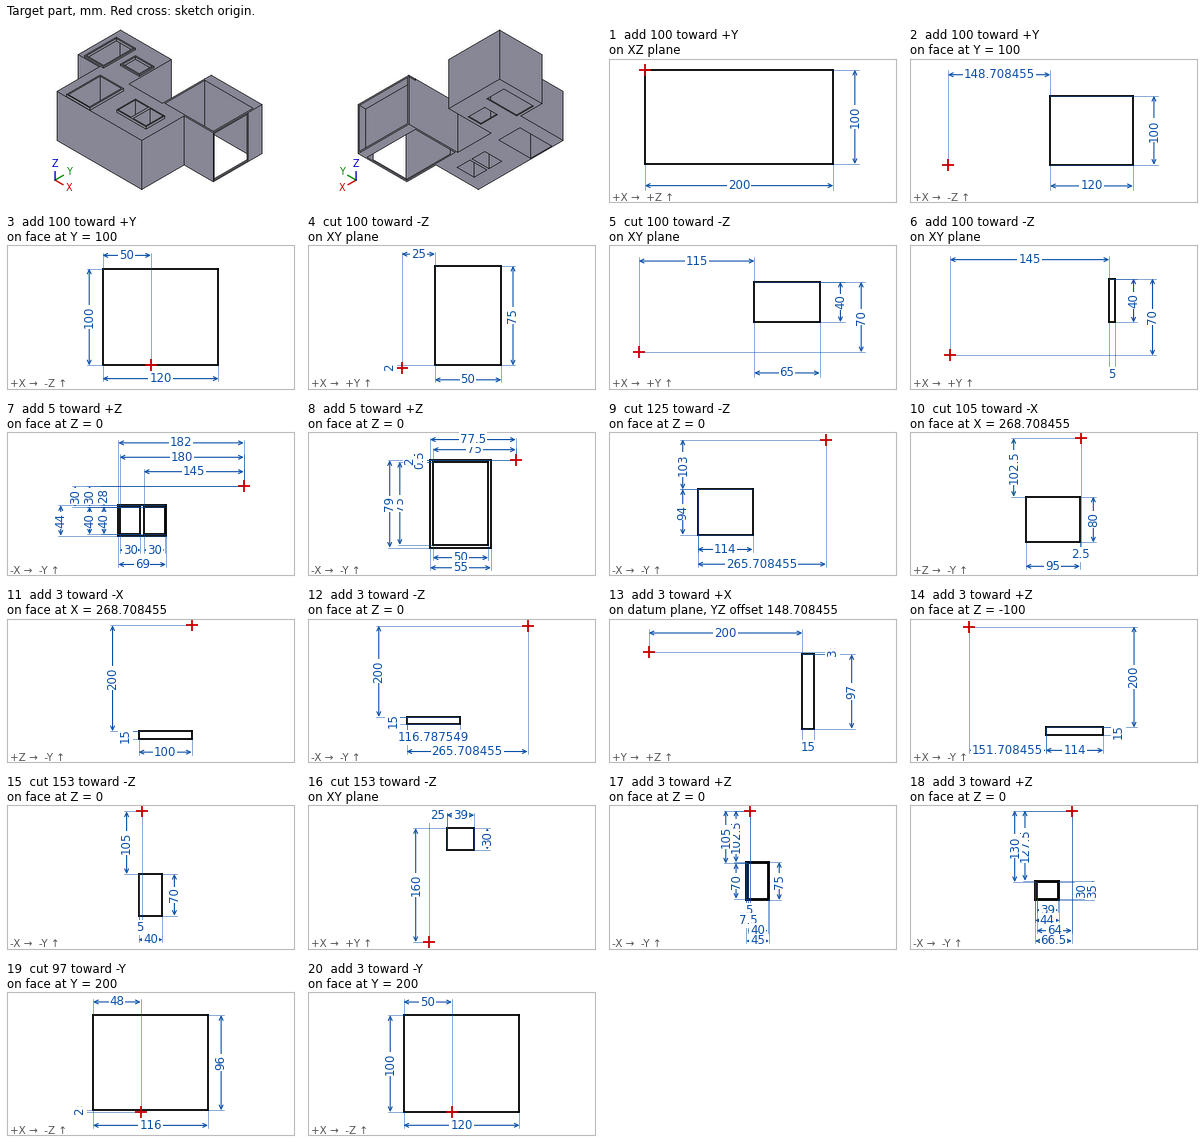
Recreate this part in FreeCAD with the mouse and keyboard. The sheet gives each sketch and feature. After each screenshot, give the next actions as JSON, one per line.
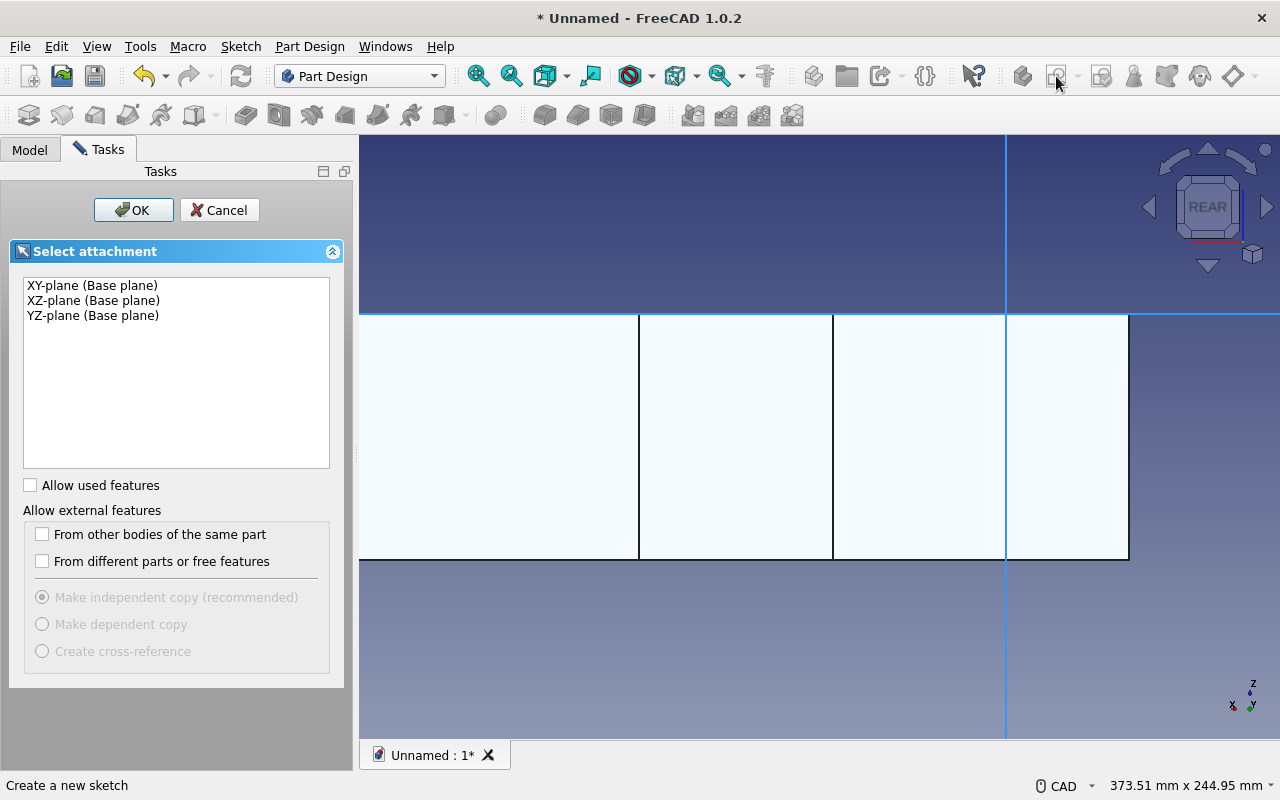
{"action": "left_click", "coordinate": [84, 286]}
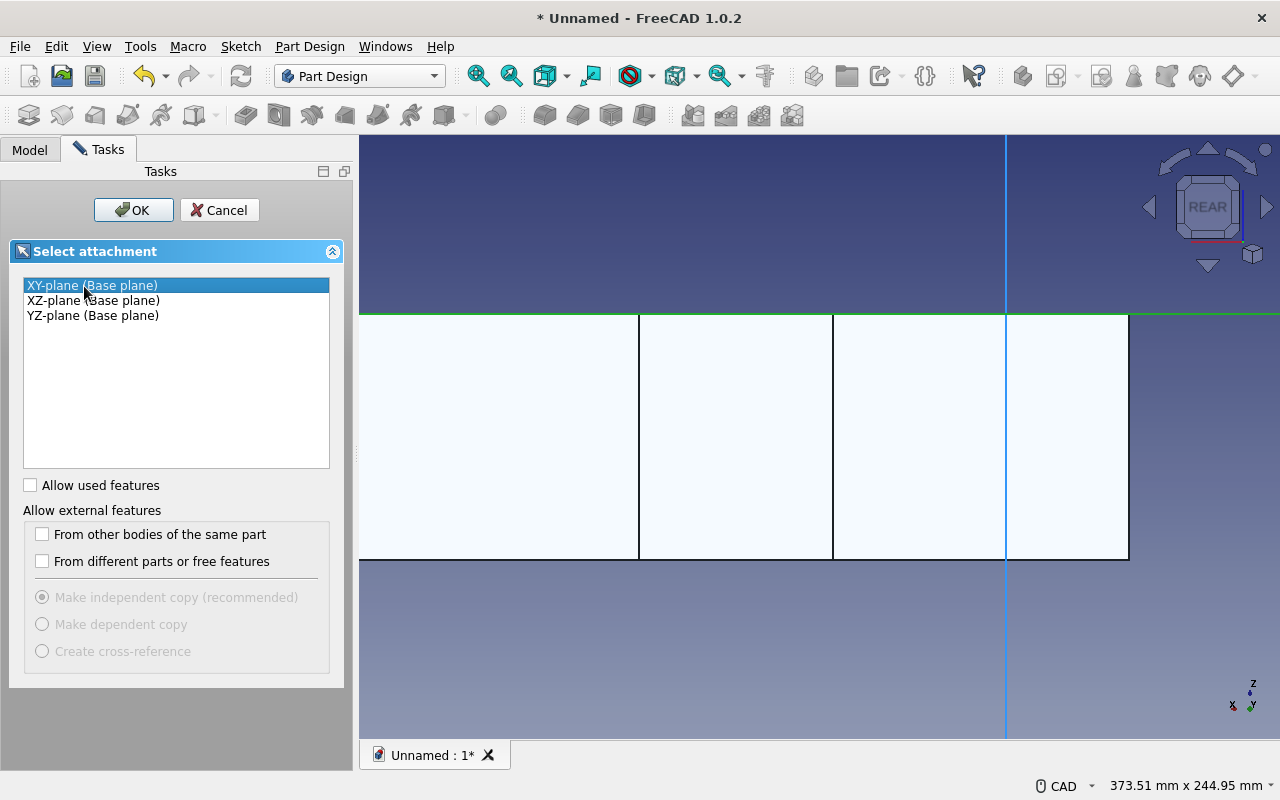
{"action": "left_click", "coordinate": [134, 210]}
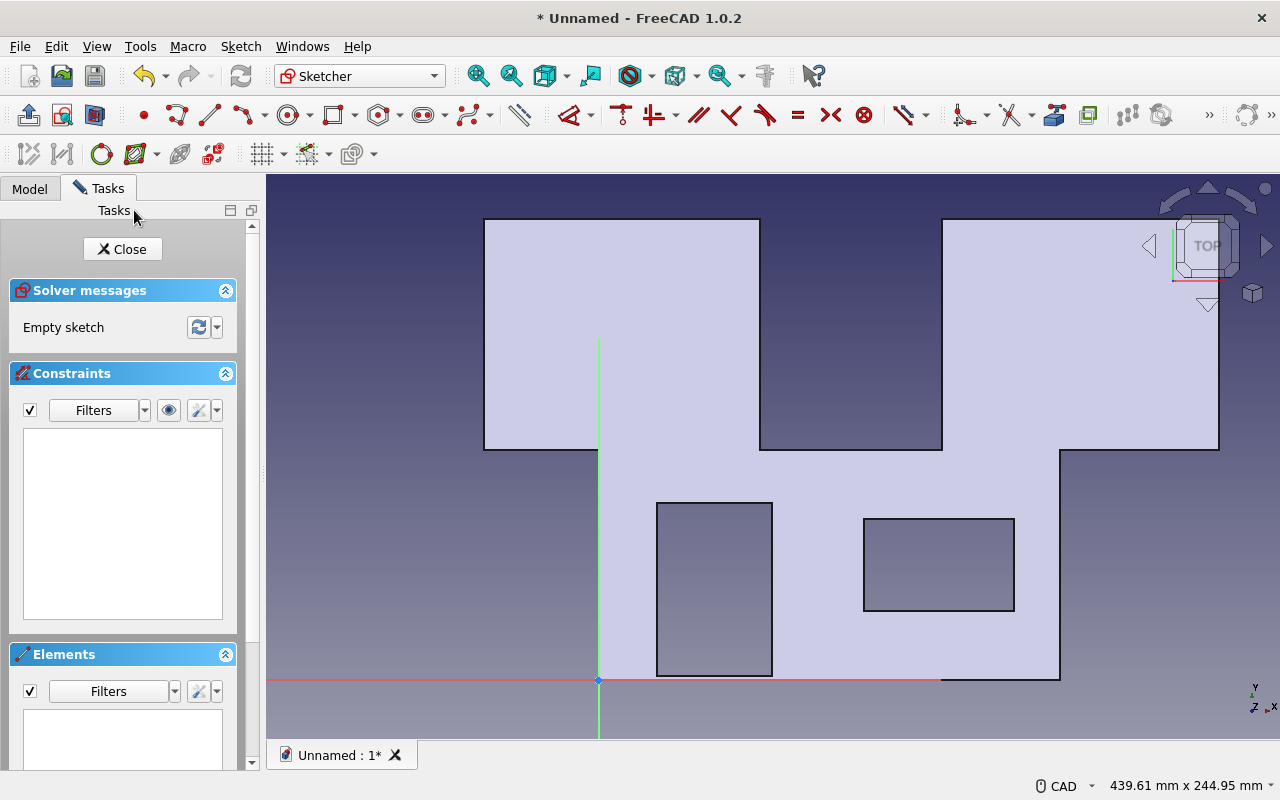
{"action": "scroll", "coordinate": [1016, 600], "scroll_direction": "up", "scroll_amount": 7}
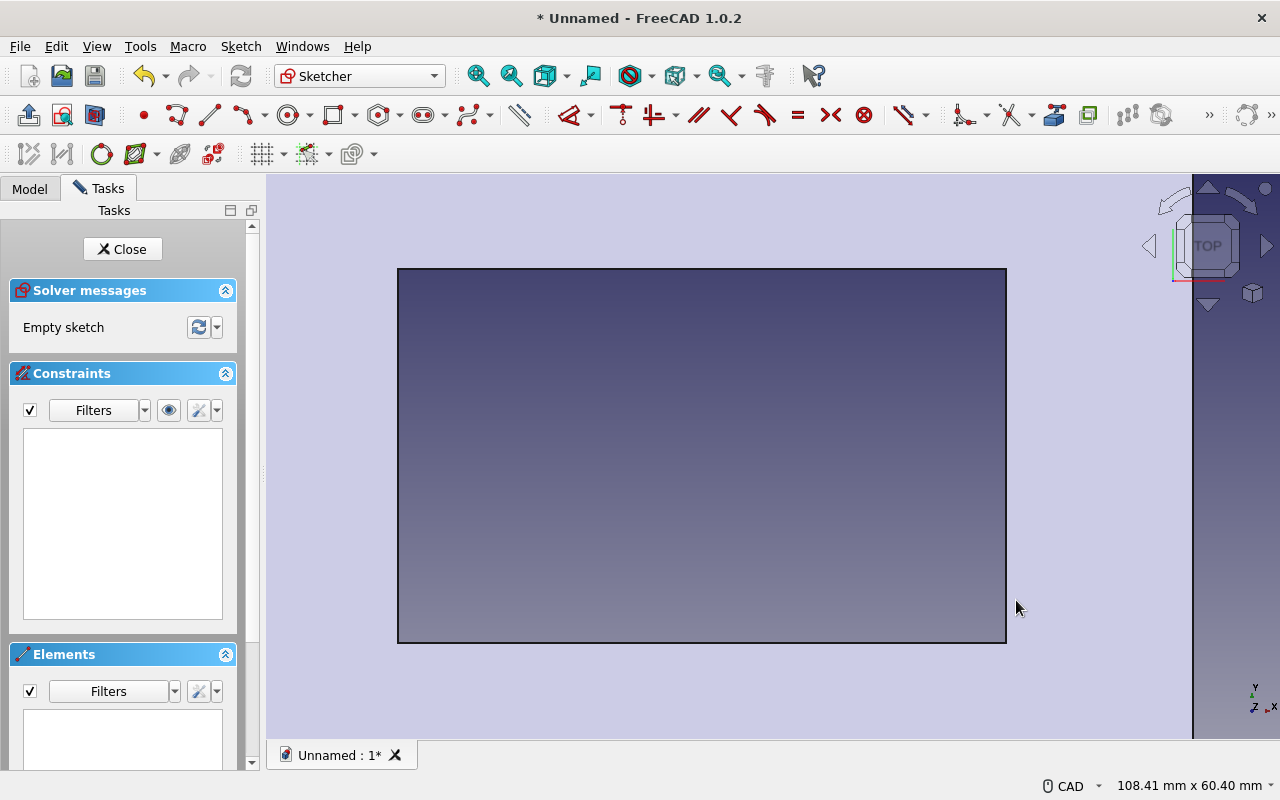
{"action": "left_click", "coordinate": [332, 116]}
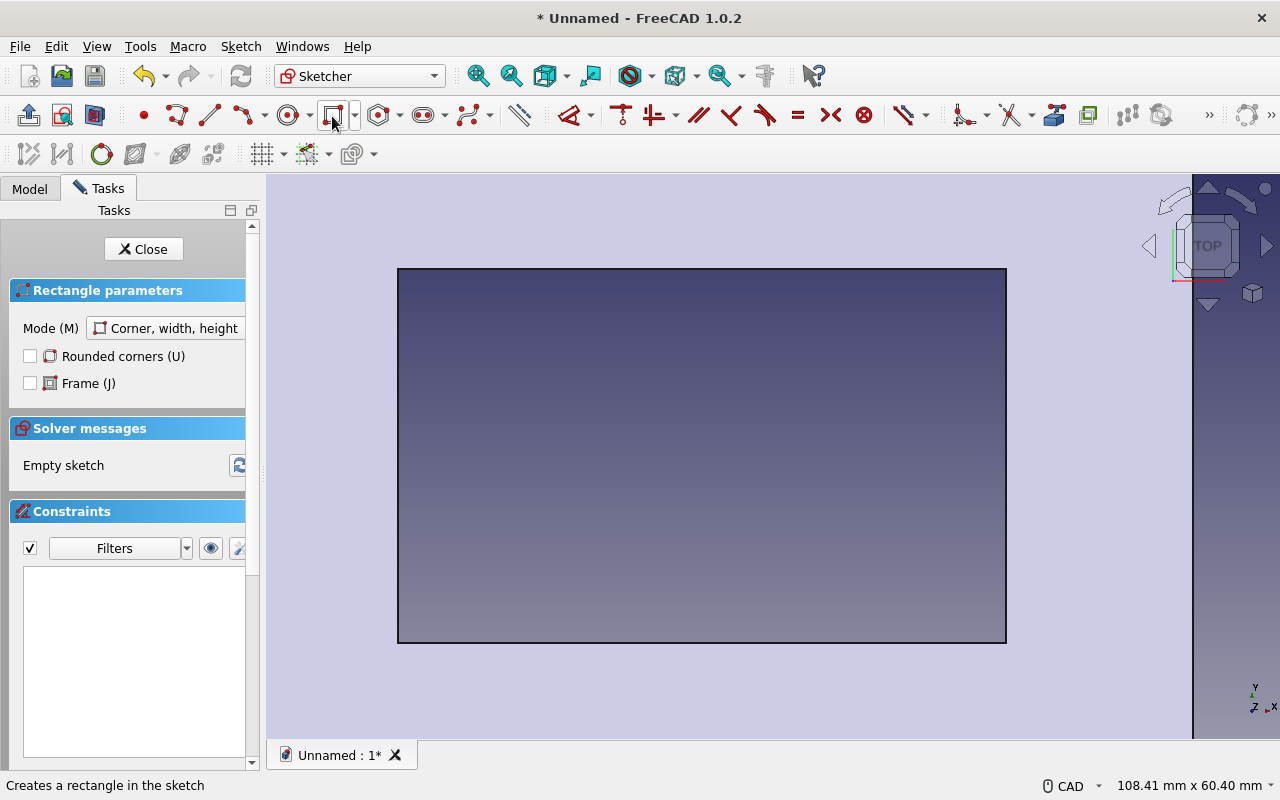
{"action": "left_click", "coordinate": [679, 269]}
{"action": "mouse_move", "coordinate": [725, 643]}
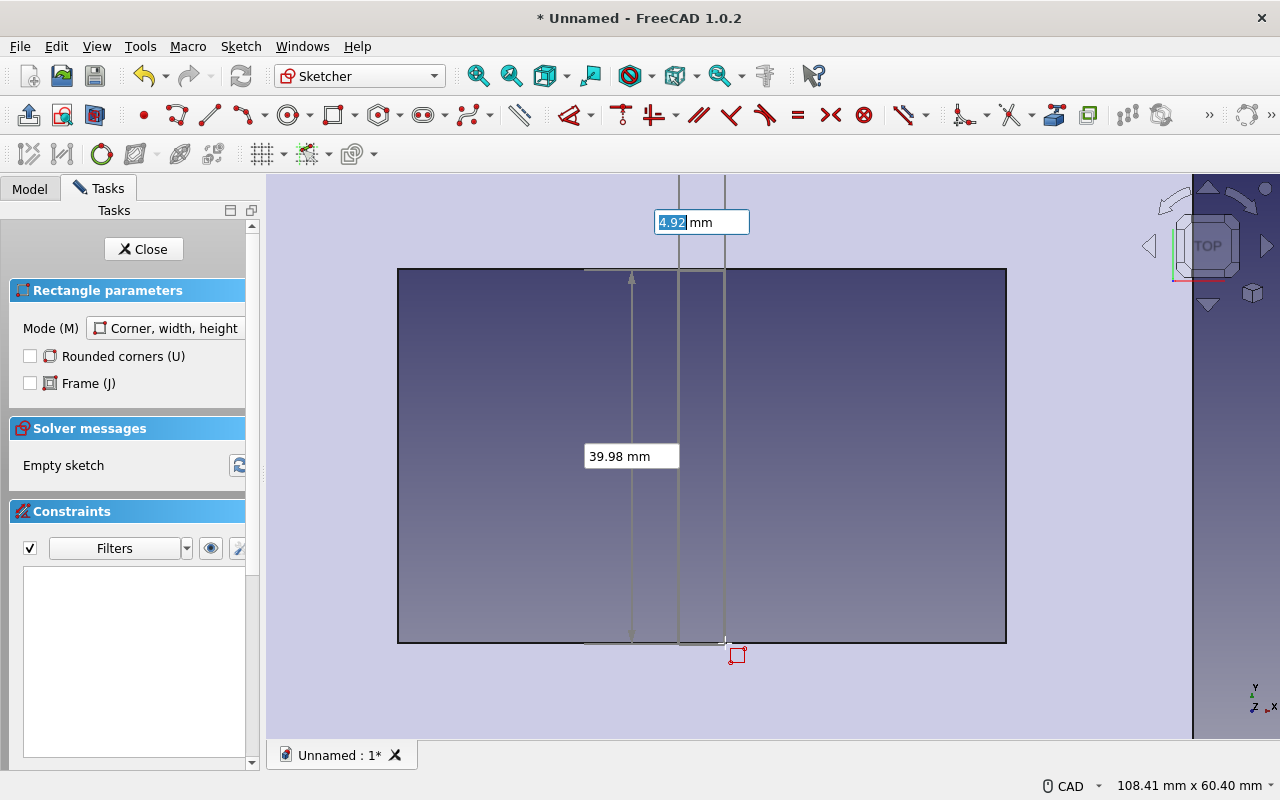
{"action": "type", "text": "5"}
{"action": "key", "text": "Tab"}
{"action": "type", "text": "40"}
{"action": "key", "text": "Return"}
{"action": "key", "text": "Escape"}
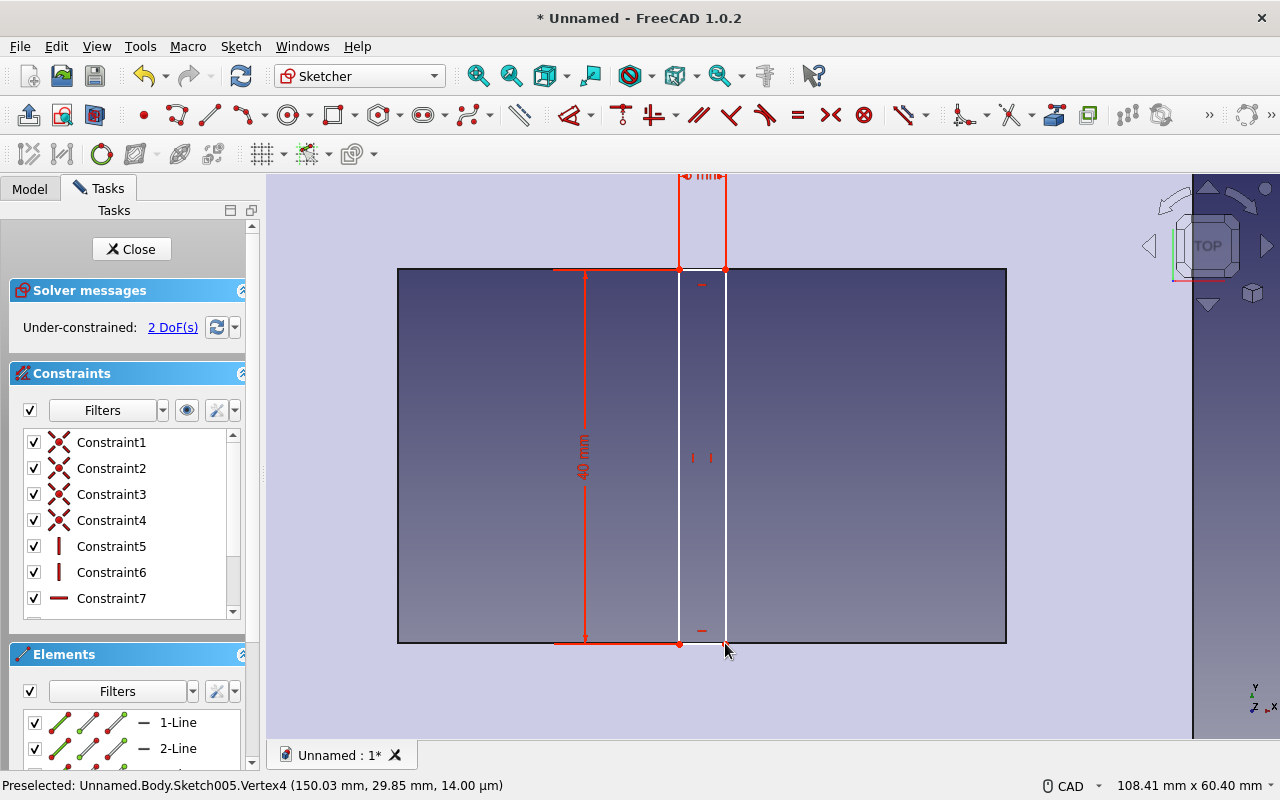
{"action": "left_click", "coordinate": [568, 116]}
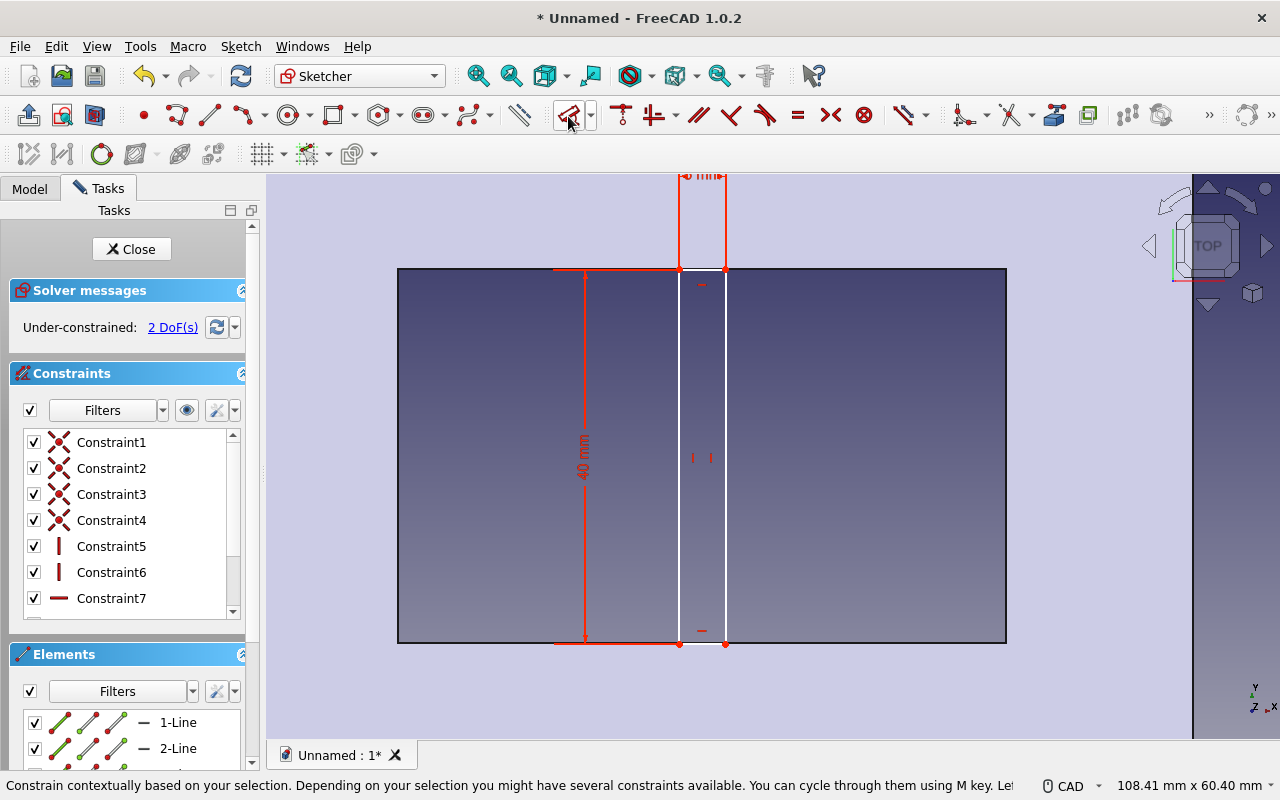
{"action": "left_click", "coordinate": [679, 270]}
{"action": "left_click", "coordinate": [761, 491]}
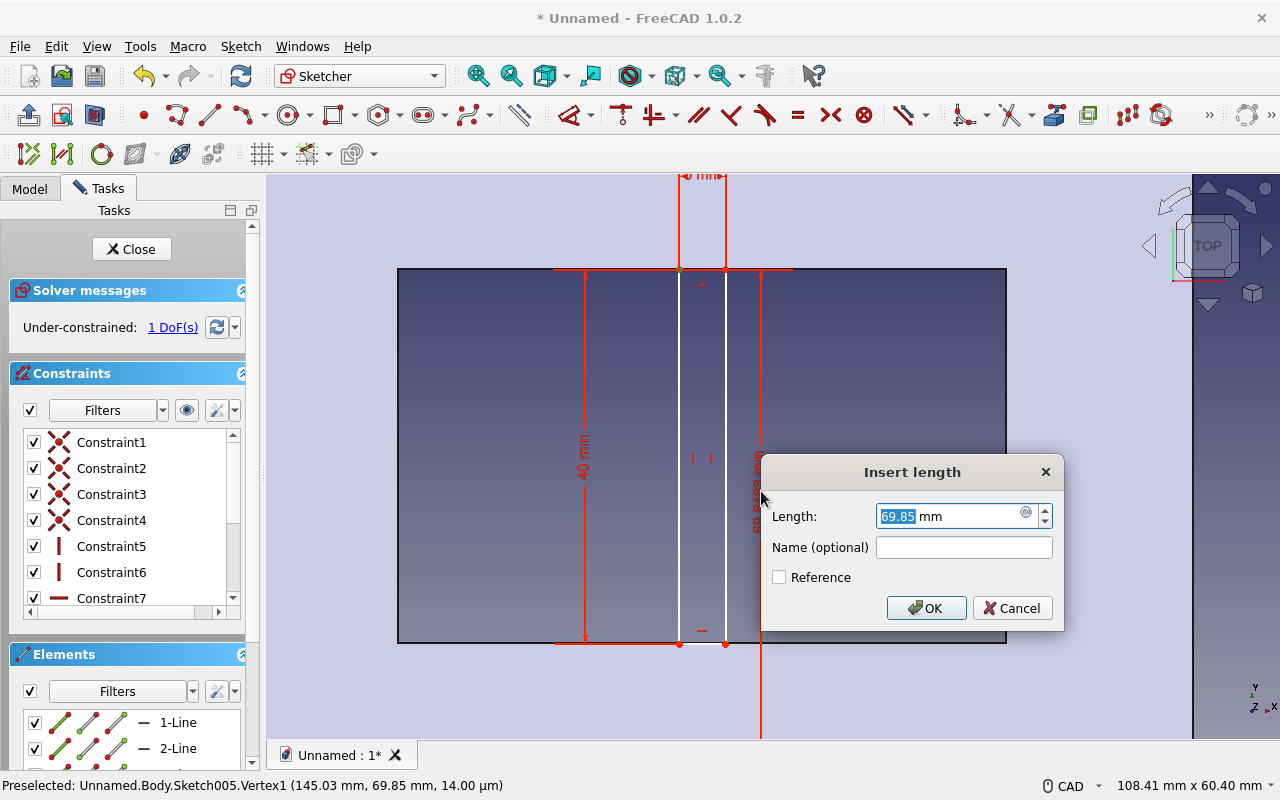
{"action": "type", "text": "70"}
{"action": "key", "text": "Return"}